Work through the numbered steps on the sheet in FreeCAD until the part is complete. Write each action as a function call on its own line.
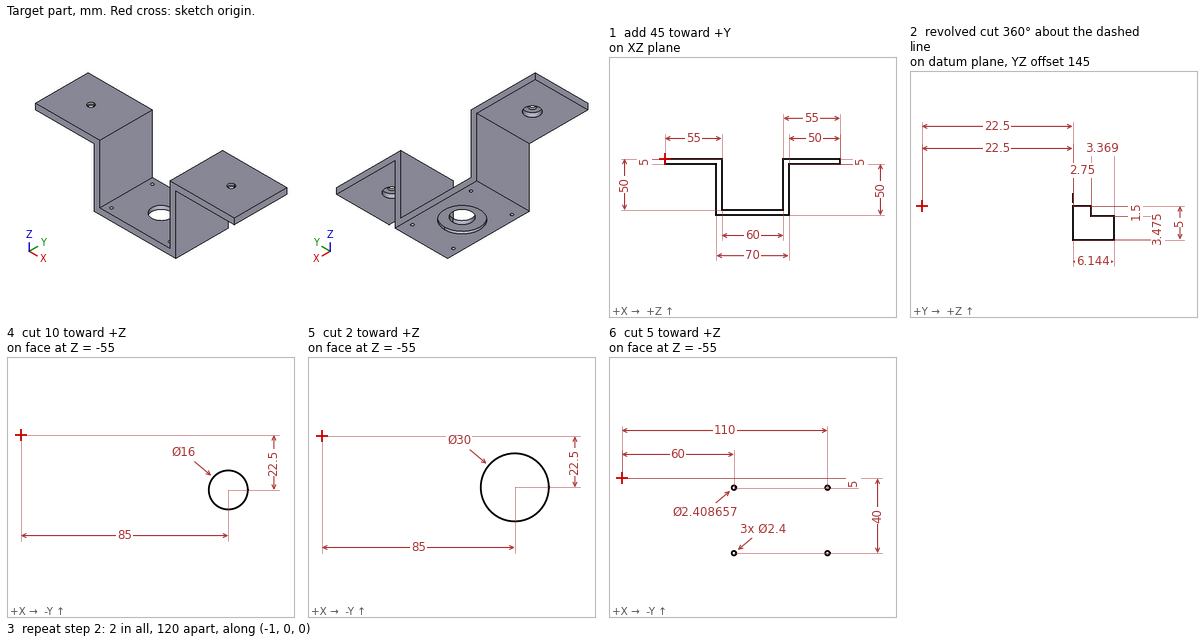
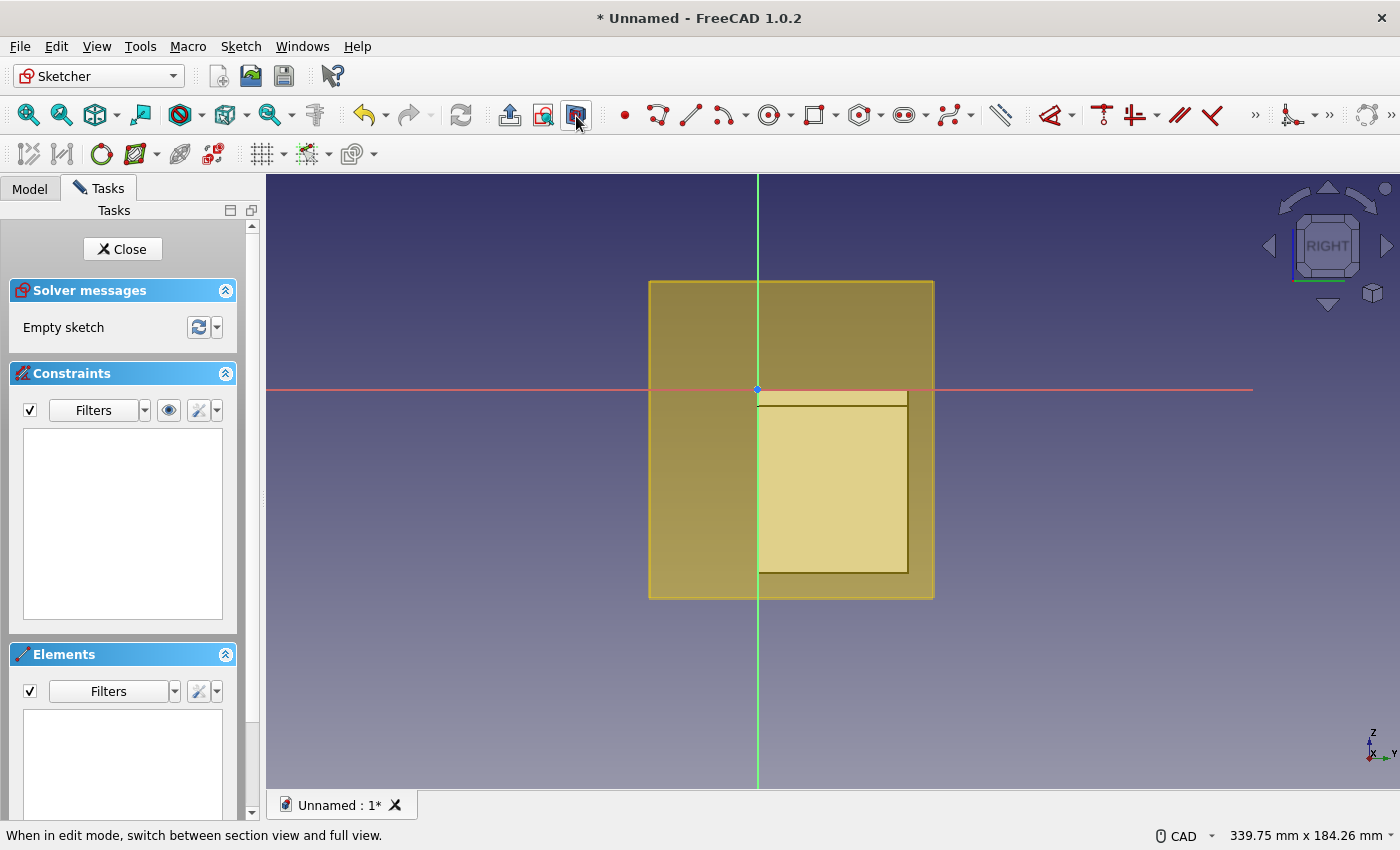
scroll(848, 389, up, 14)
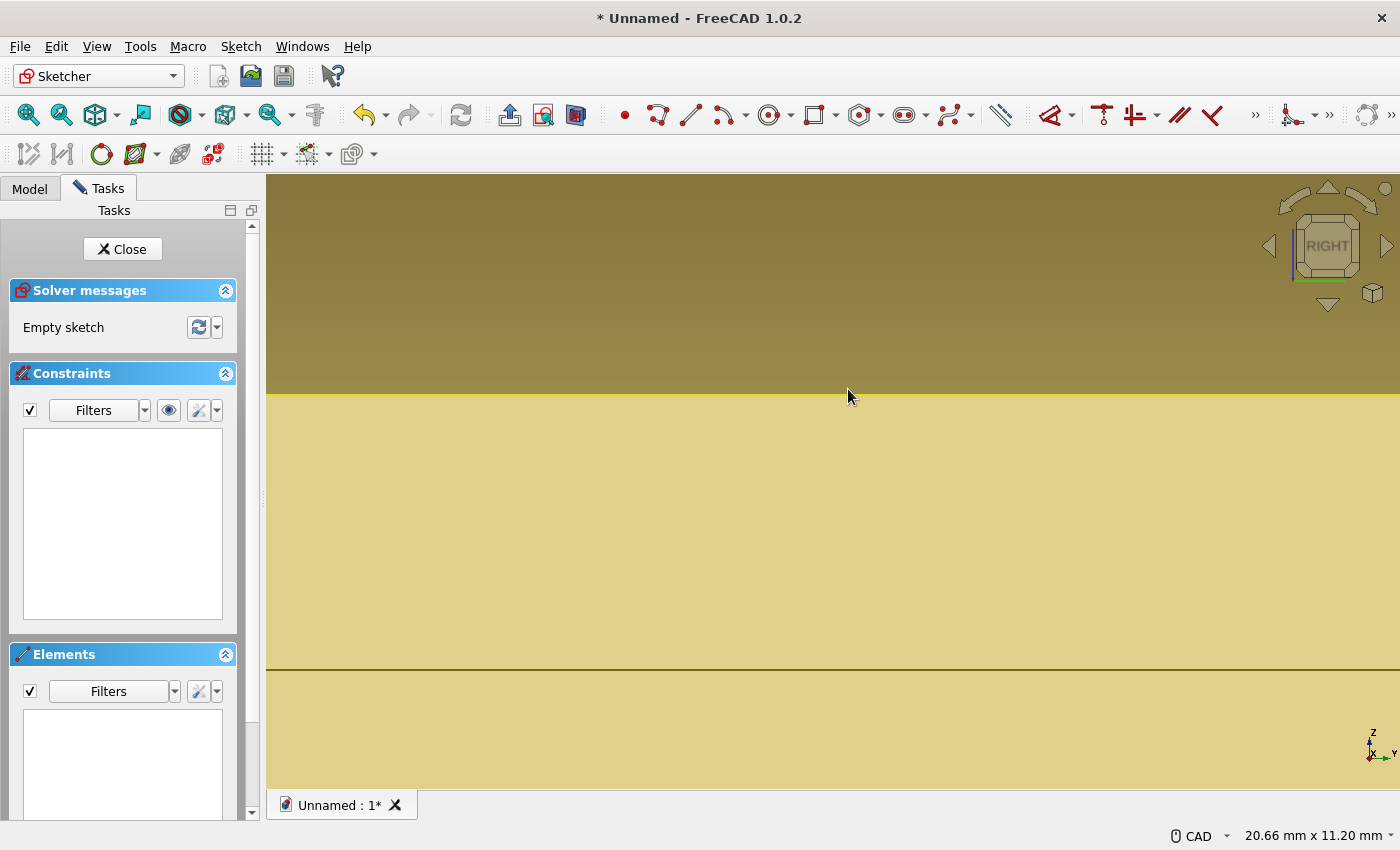
click(658, 116)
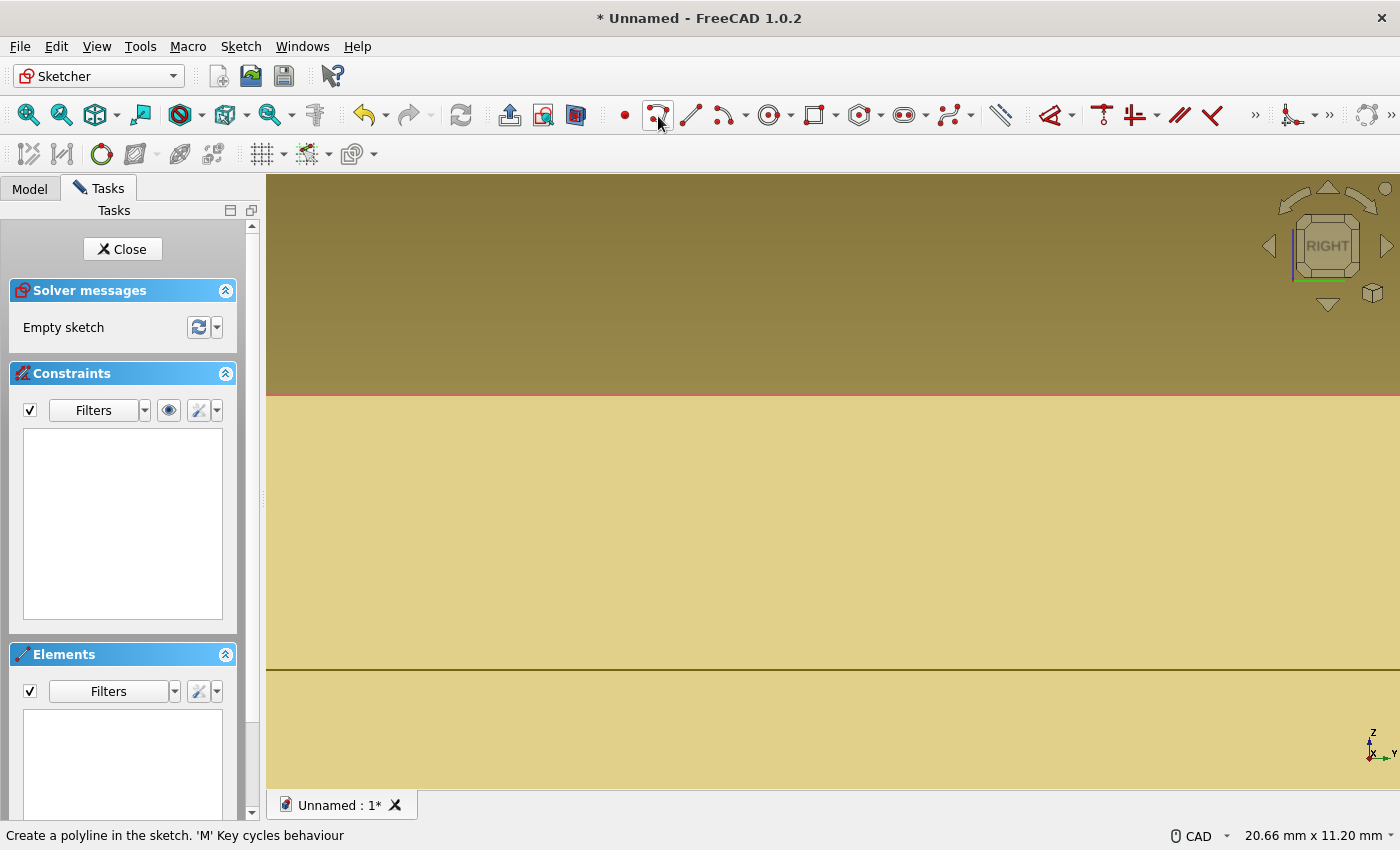
click(593, 395)
click(593, 670)
click(931, 670)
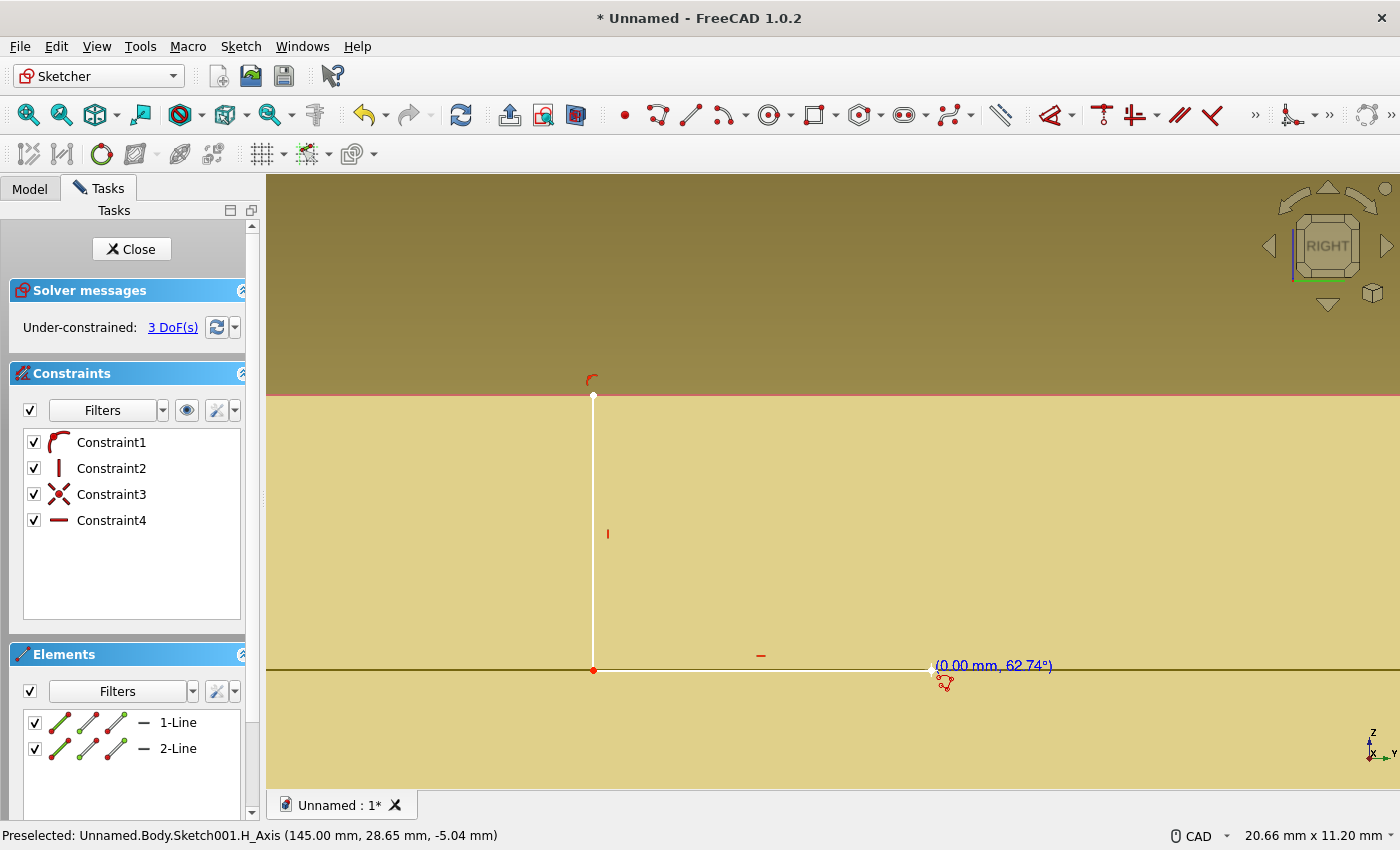
scroll(929, 668, up, 13)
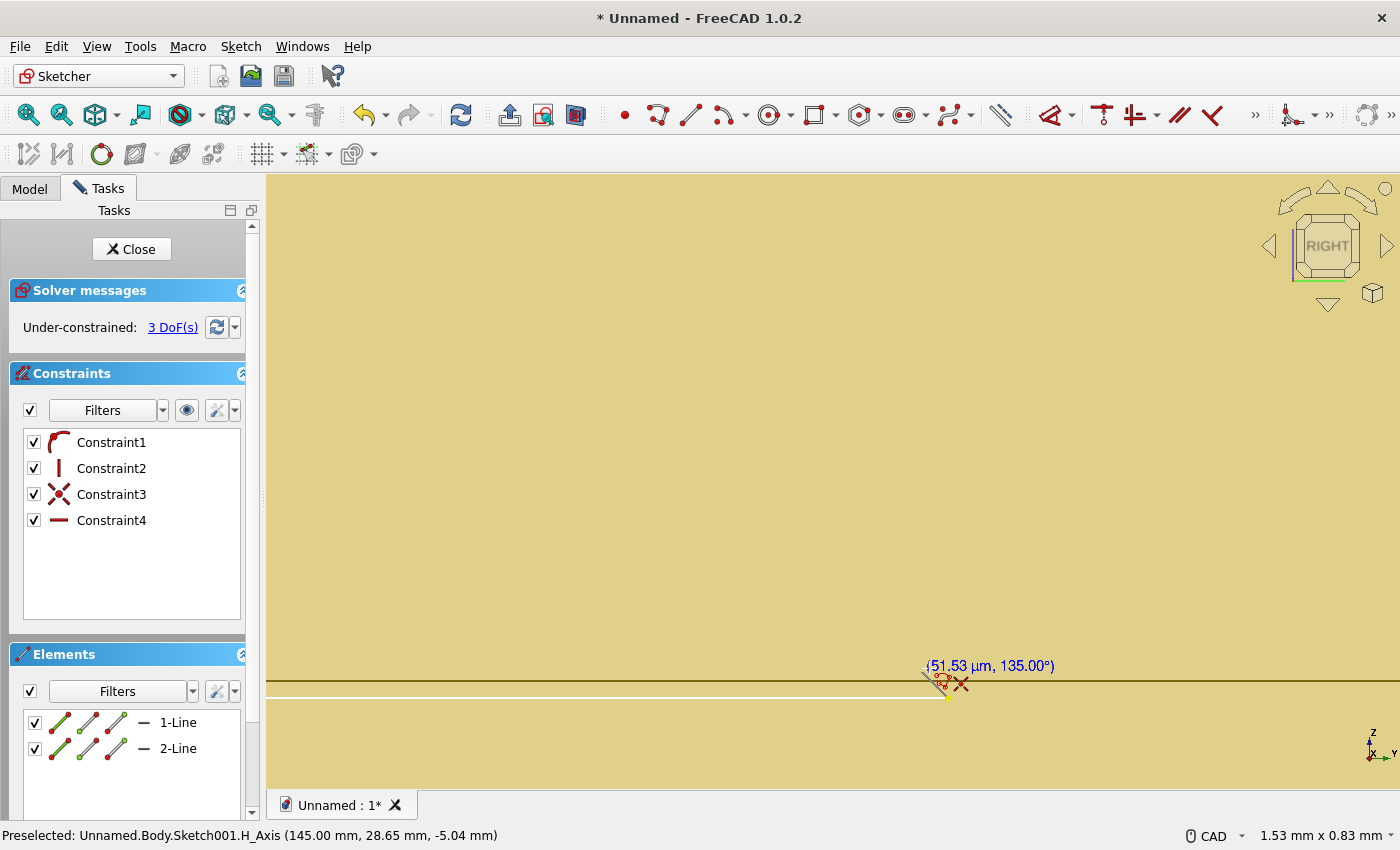
click(925, 663)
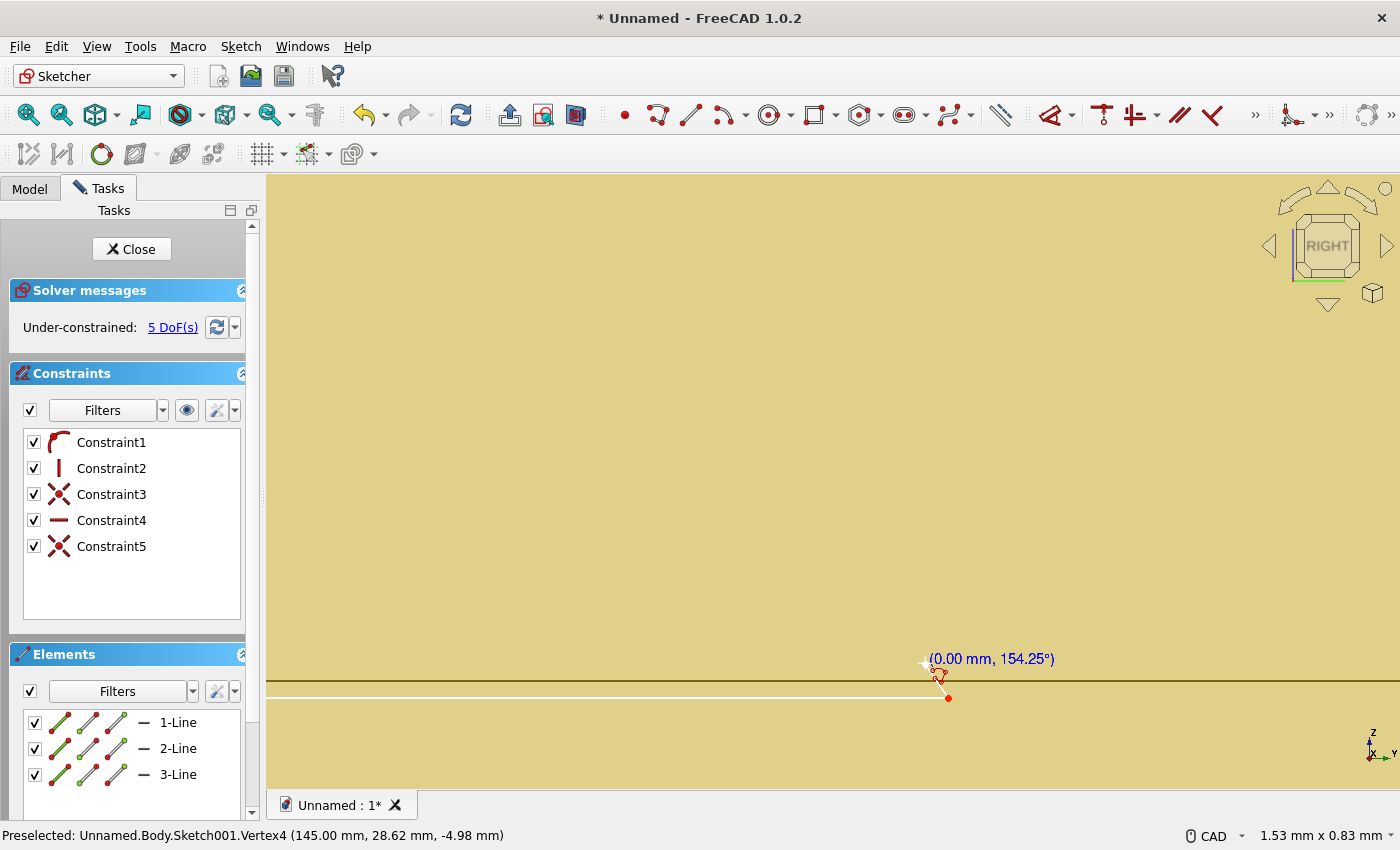
scroll(932, 673, down, 13)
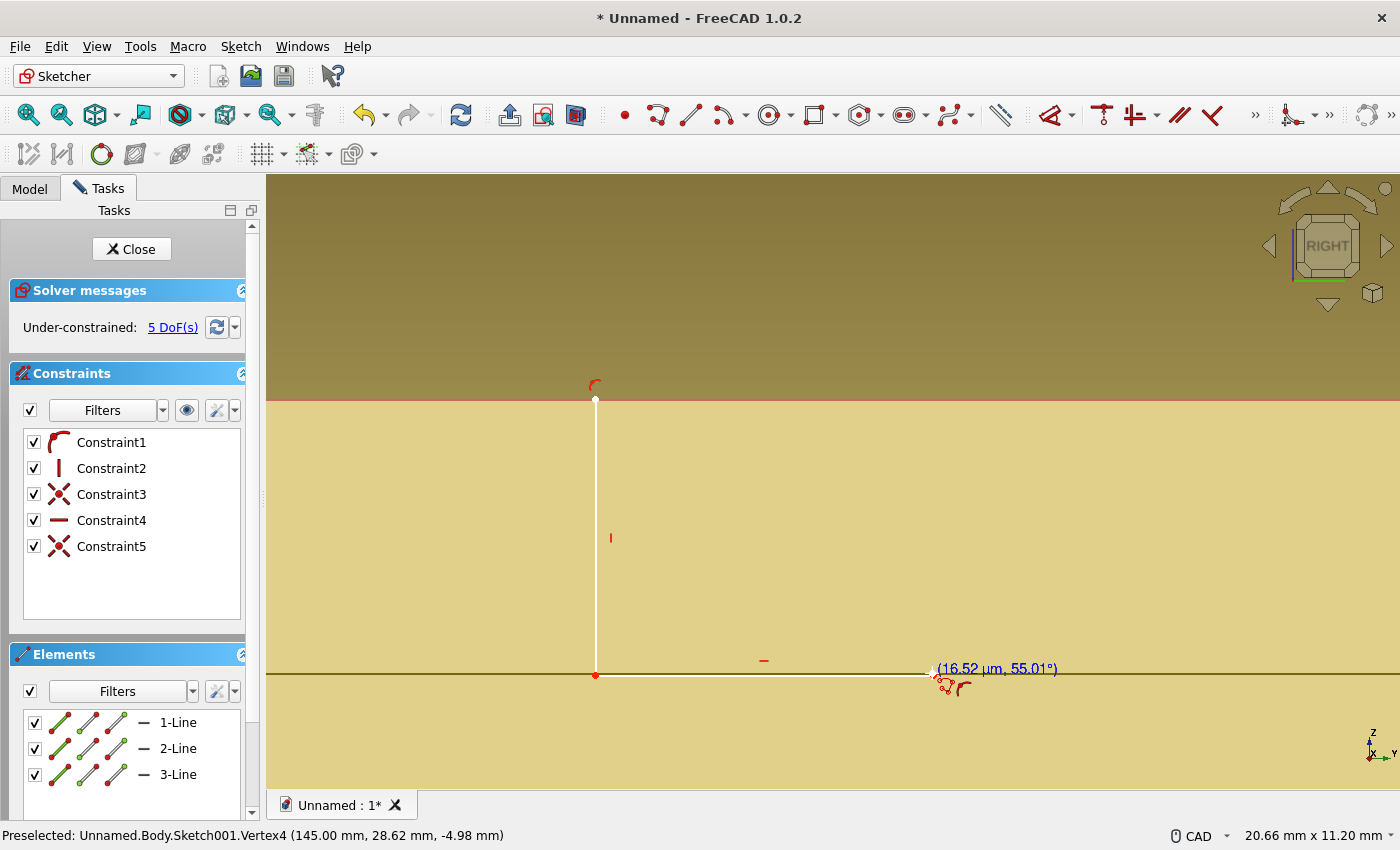
click(932, 482)
click(747, 482)
click(747, 409)
click(596, 400)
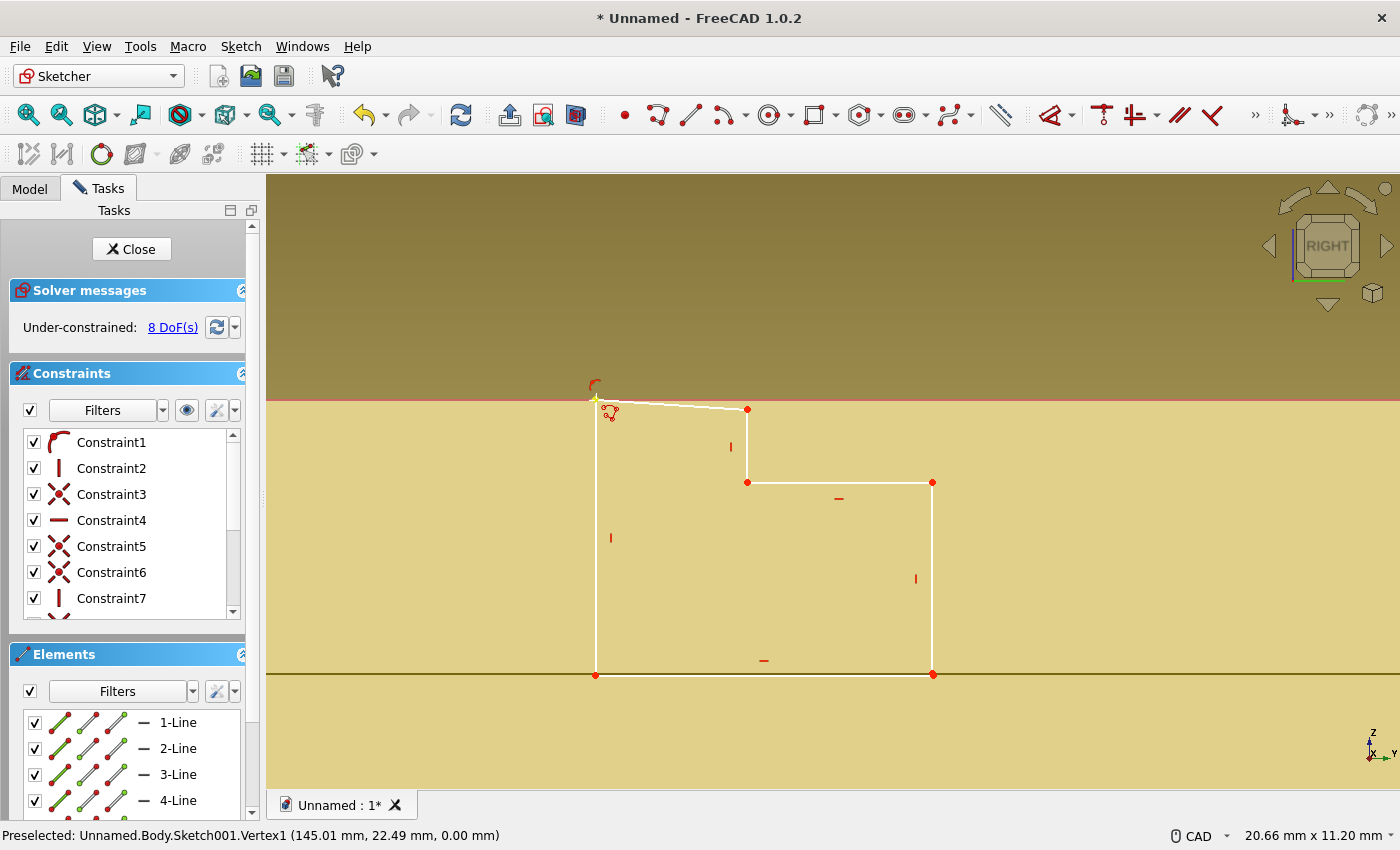
click(691, 116)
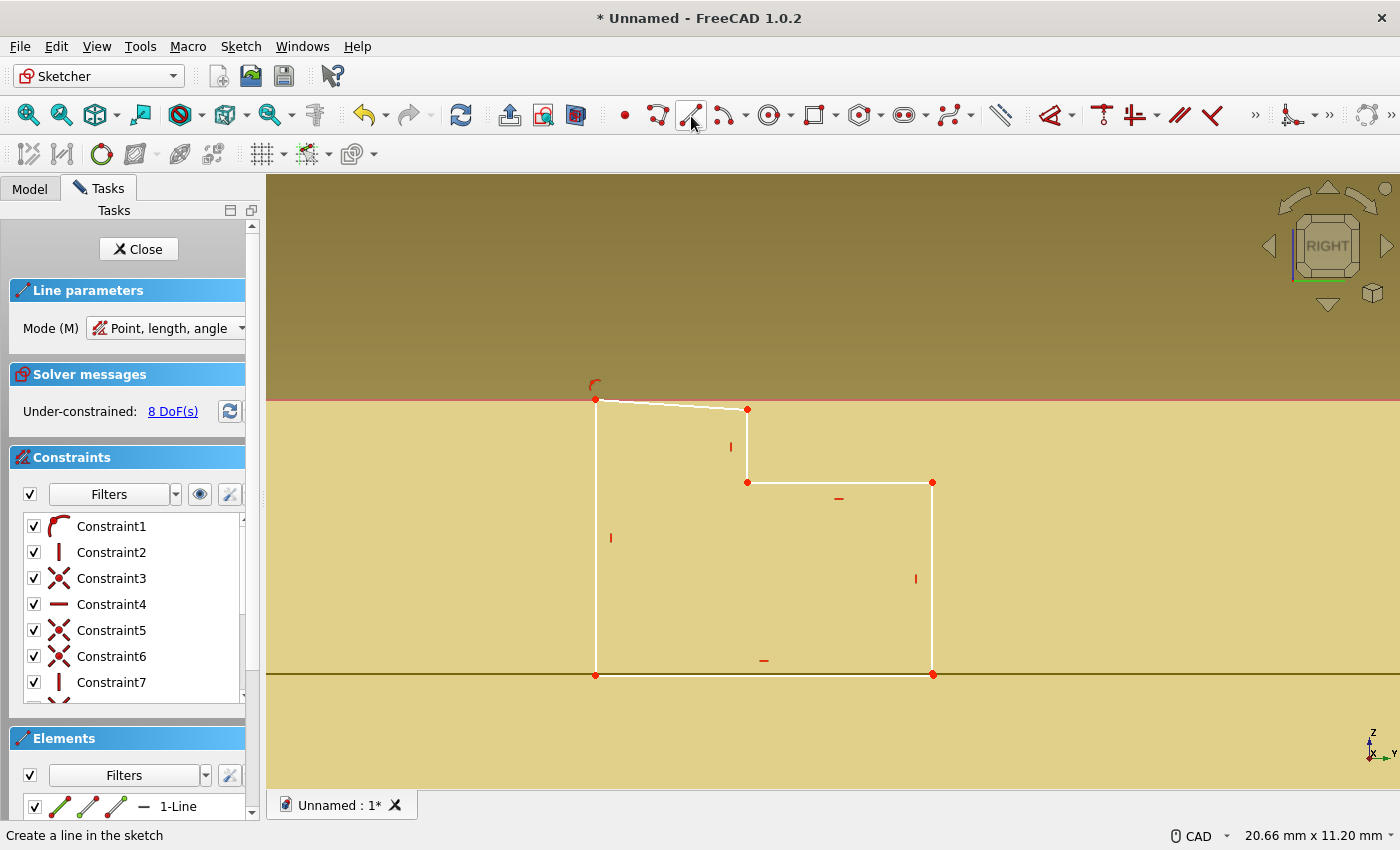
click(596, 372)
click(596, 290)
key(Escape)